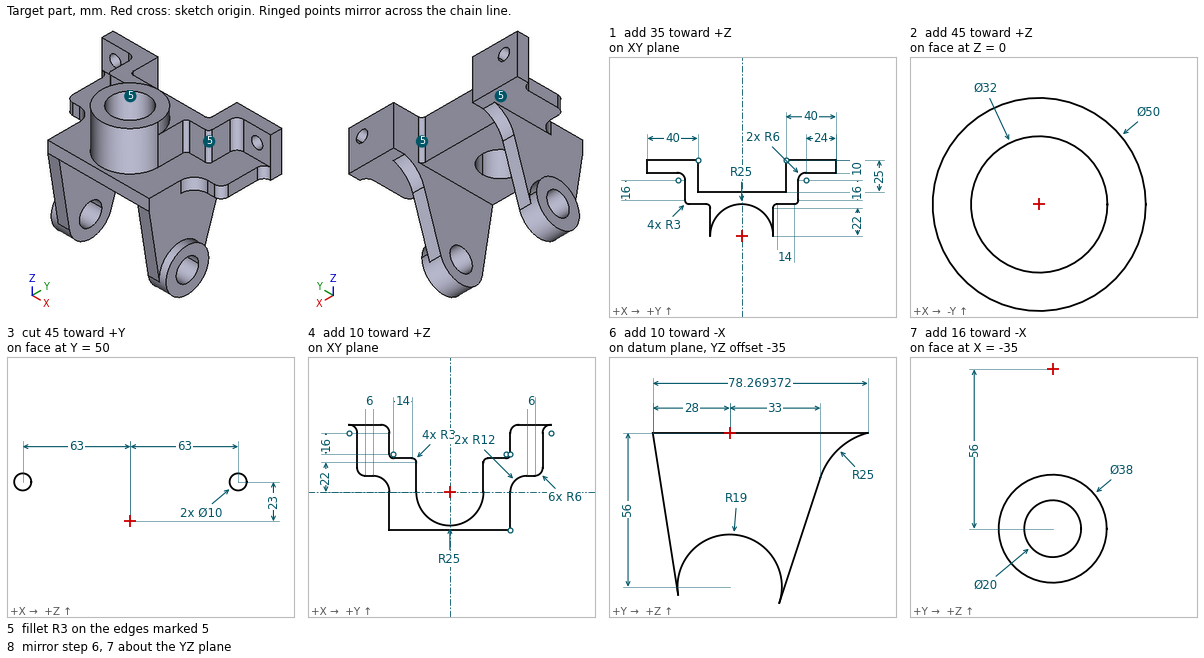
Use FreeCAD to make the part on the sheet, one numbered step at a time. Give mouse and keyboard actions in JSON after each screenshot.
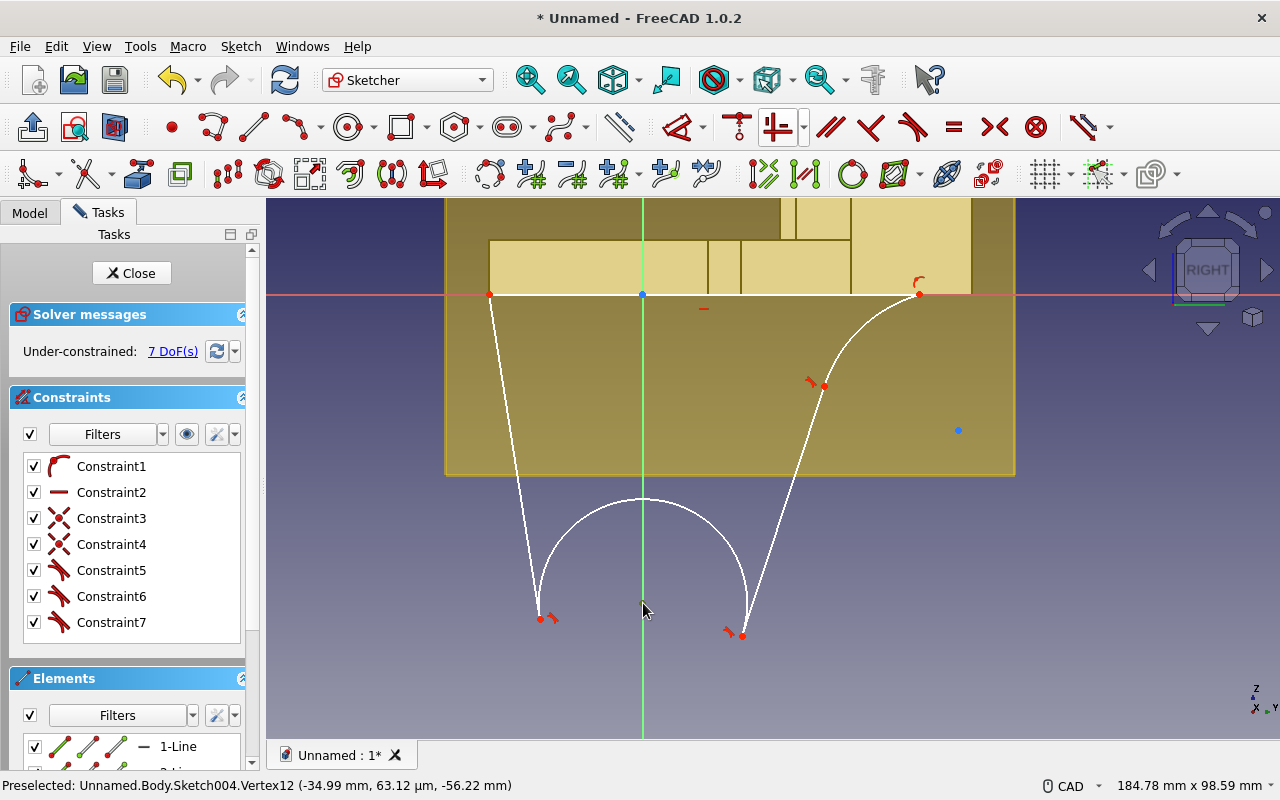
{"action": "left_click", "coordinate": [643, 676]}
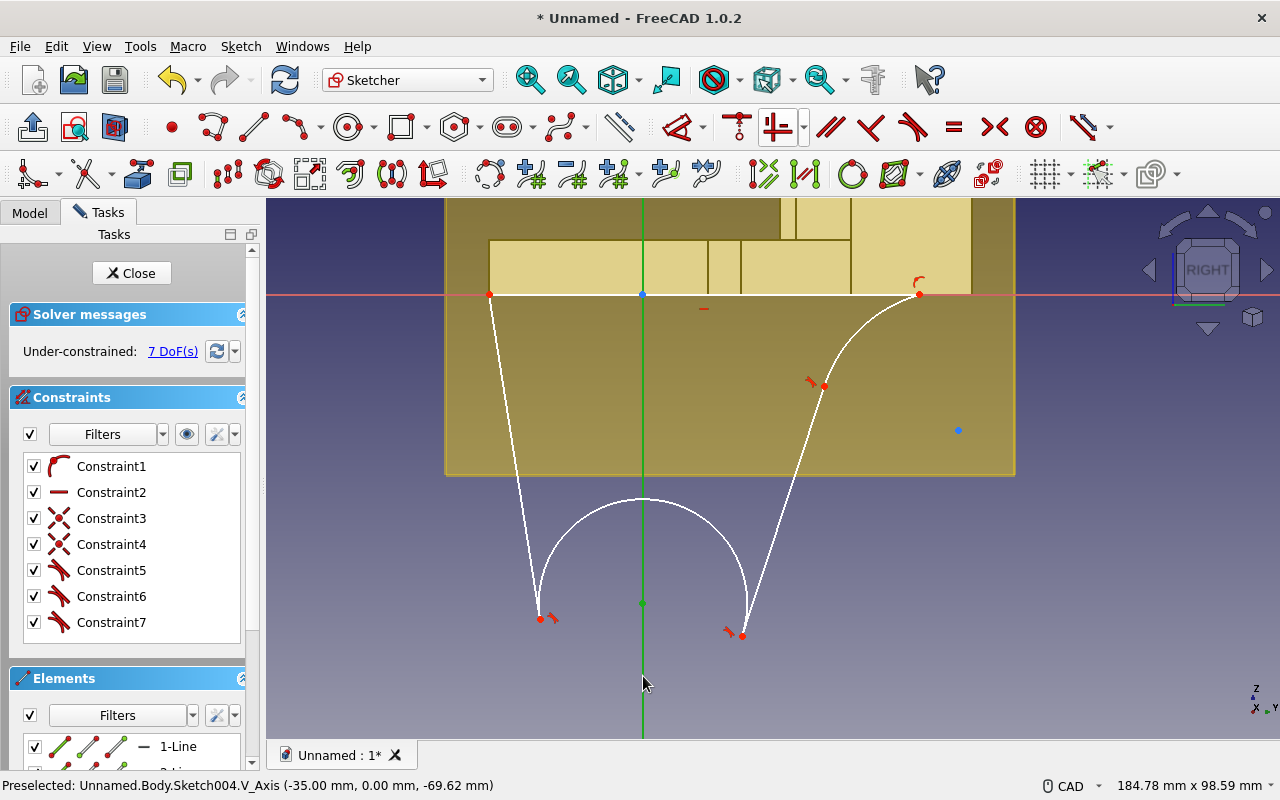
{"action": "left_click", "coordinate": [737, 128]}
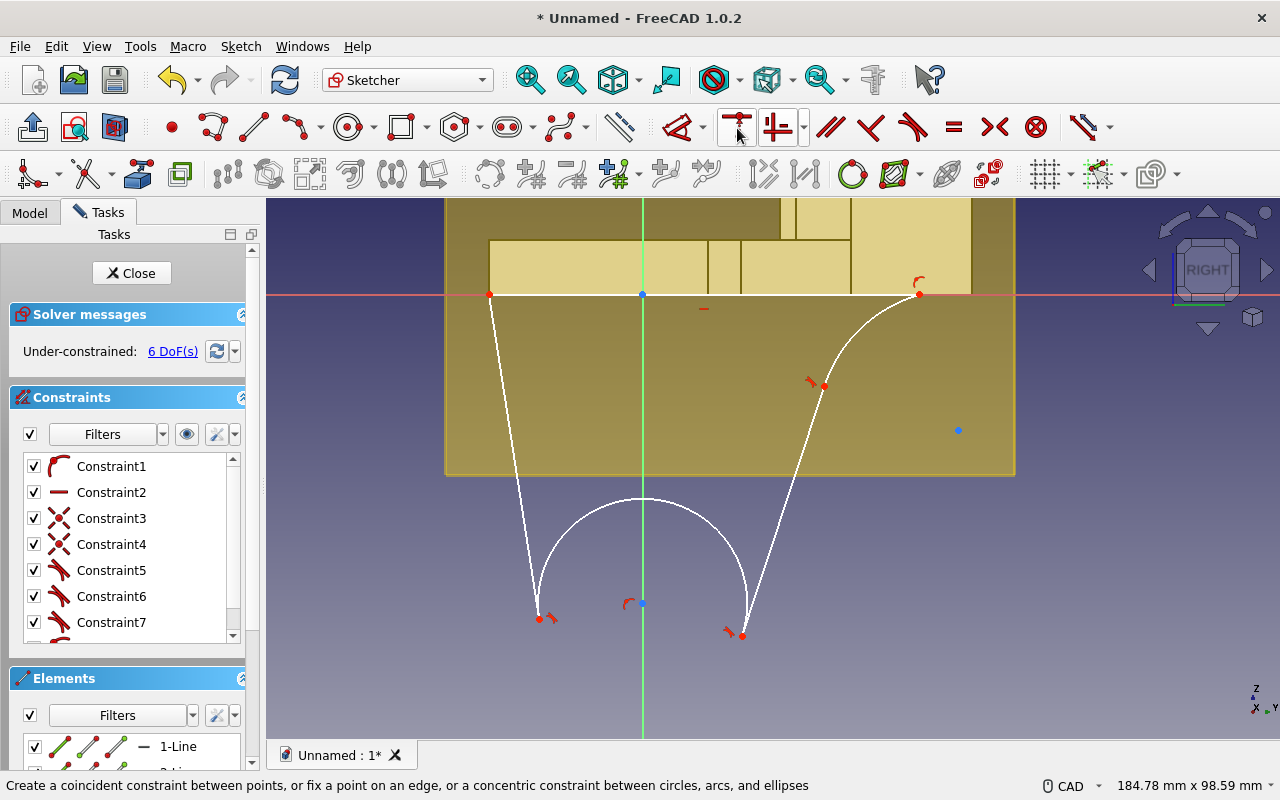
{"action": "left_click", "coordinate": [676, 128]}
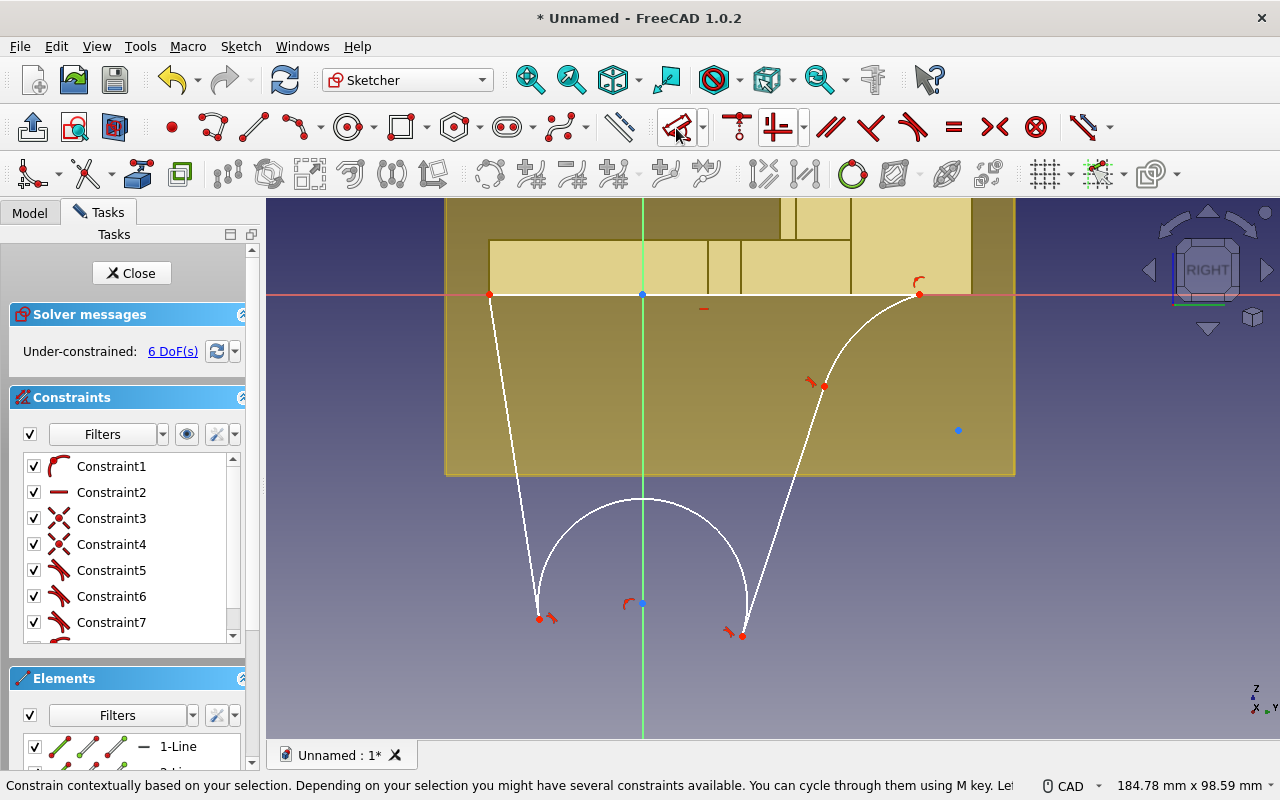
{"action": "left_click", "coordinate": [882, 312]}
{"action": "left_click", "coordinate": [946, 258]}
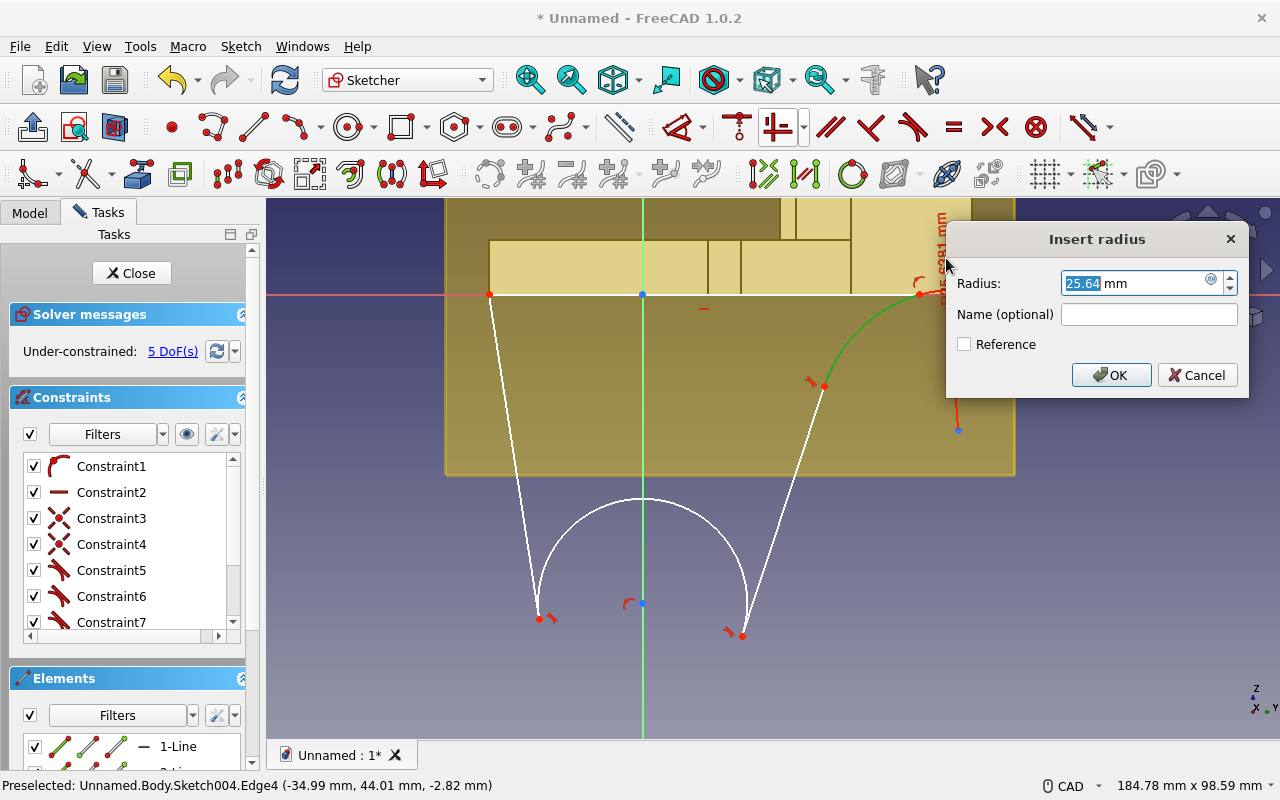
{"action": "type", "text": "25"}
{"action": "key", "text": "Return"}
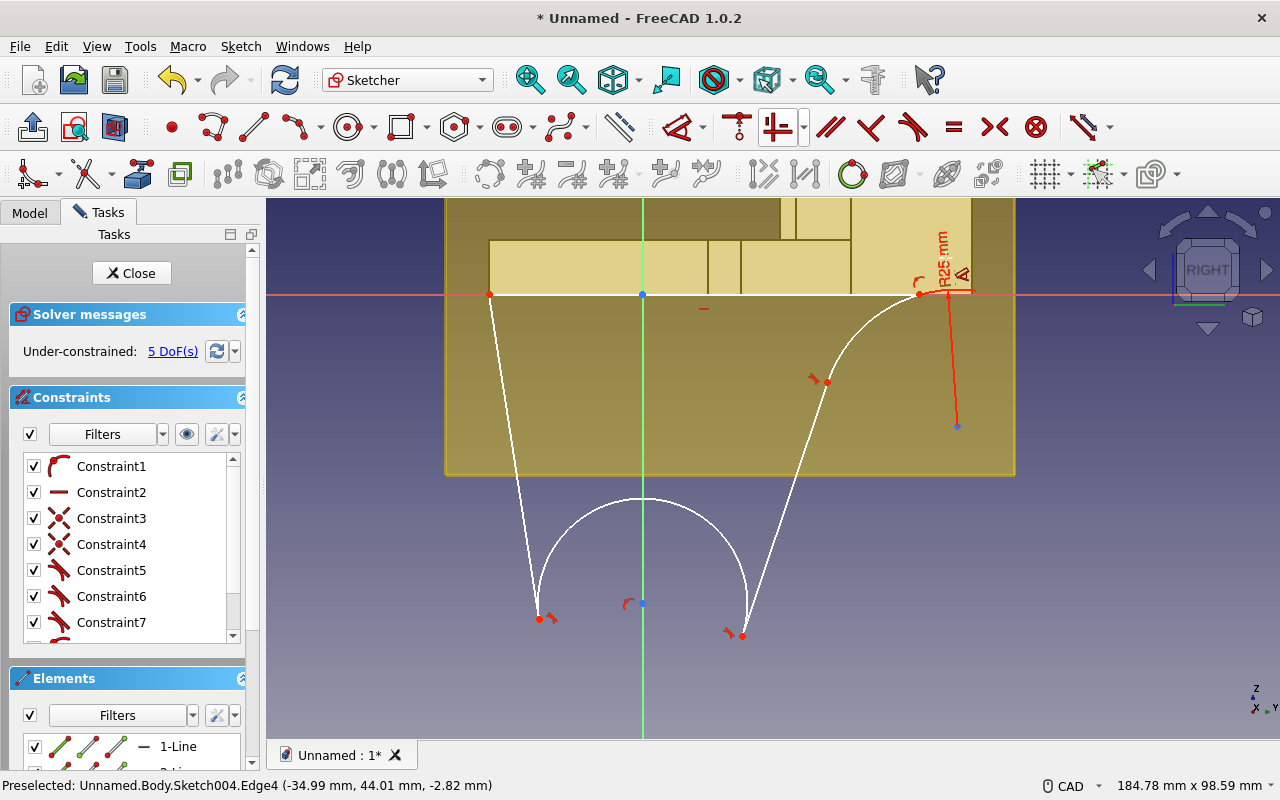
{"action": "left_click", "coordinate": [719, 531]}
{"action": "left_click", "coordinate": [742, 509]}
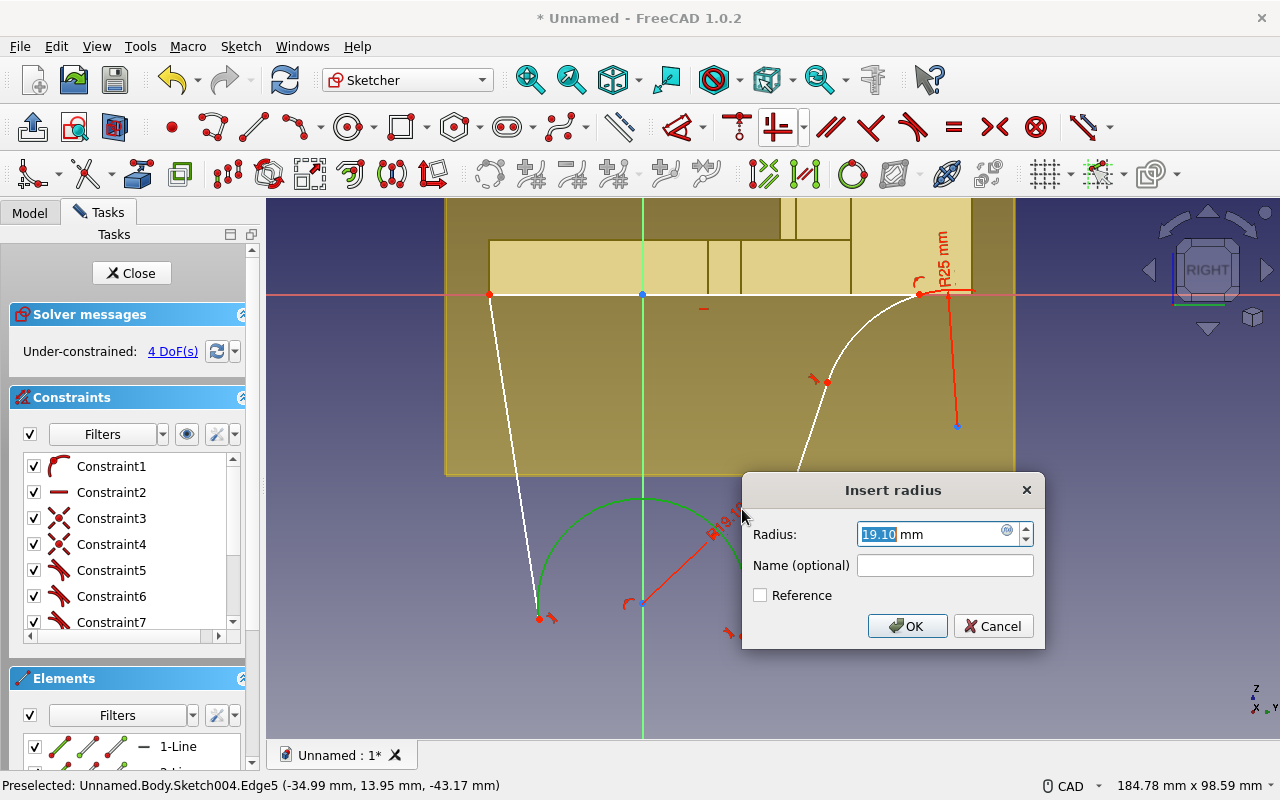
{"action": "type", "text": "19"}
{"action": "key", "text": "Return"}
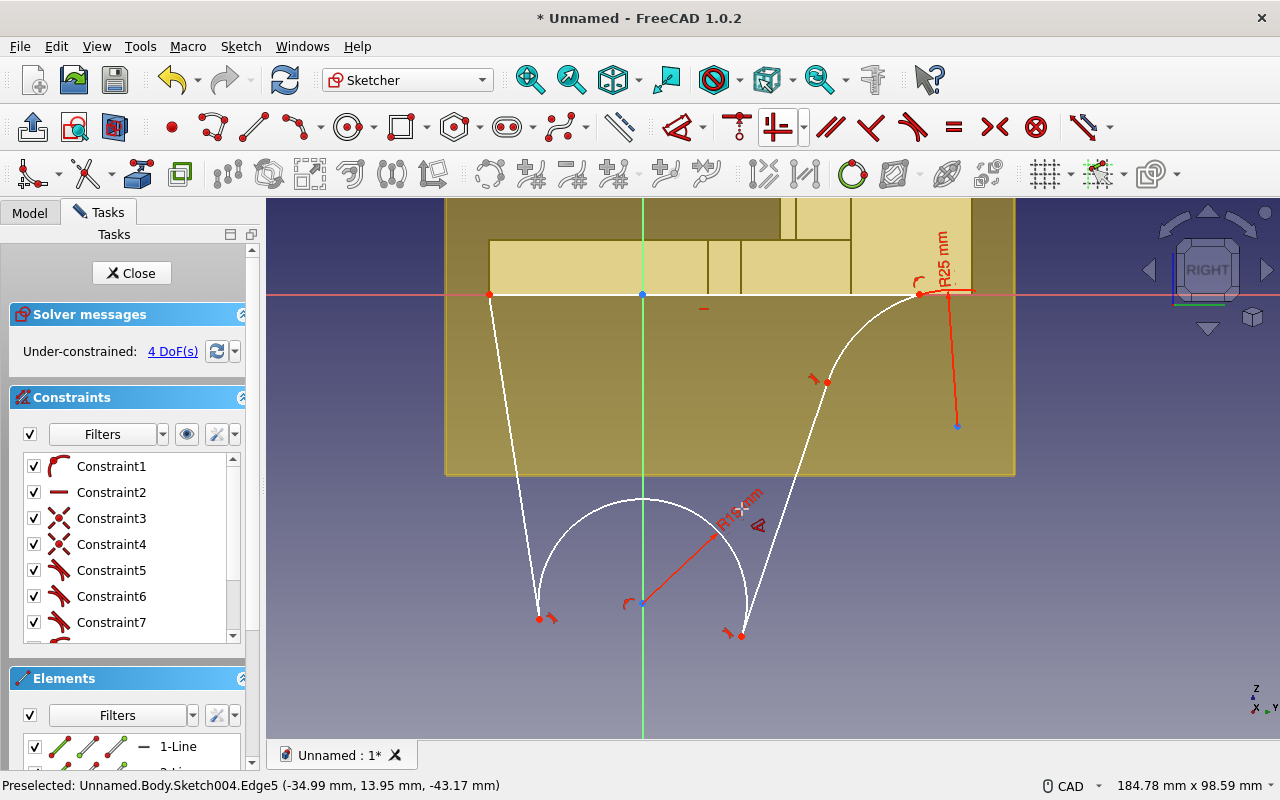
{"action": "left_click", "coordinate": [828, 383]}
{"action": "left_click", "coordinate": [735, 261]}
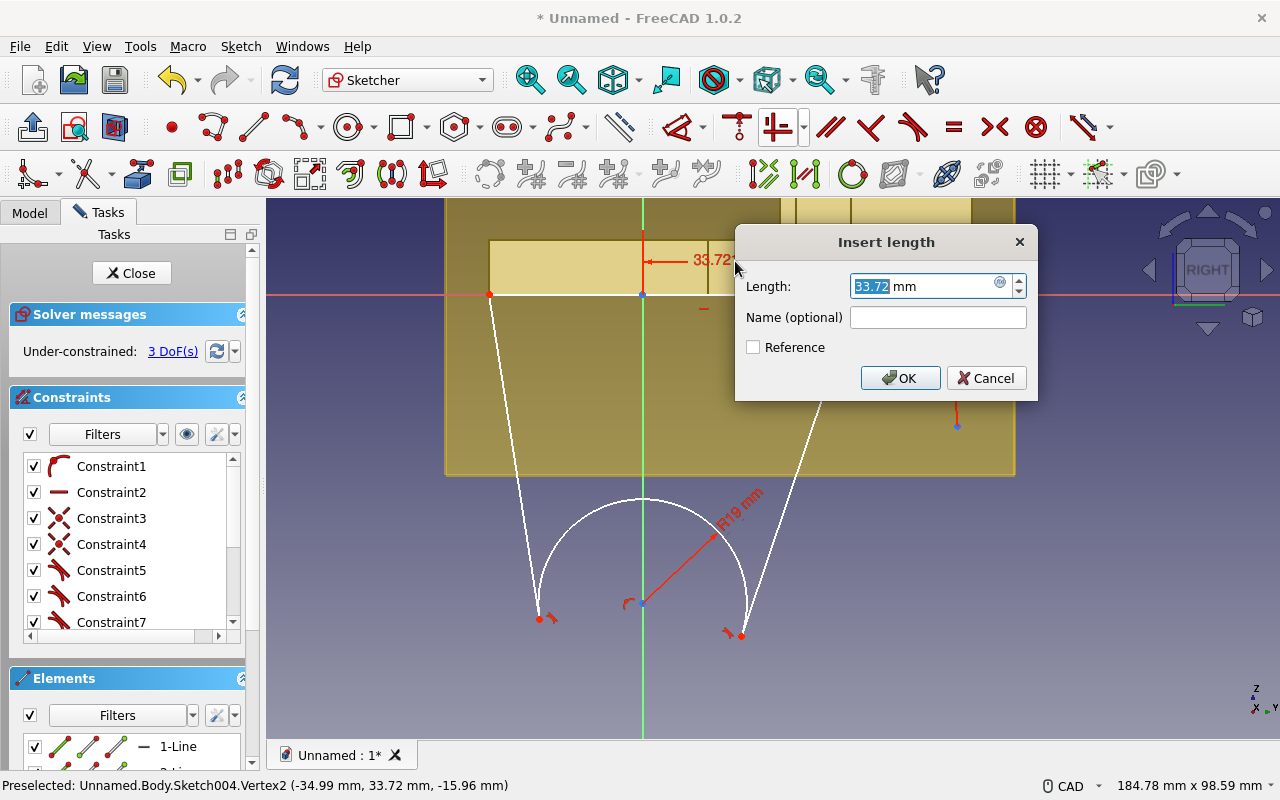
{"action": "type", "text": "33"}
{"action": "key", "text": "Return"}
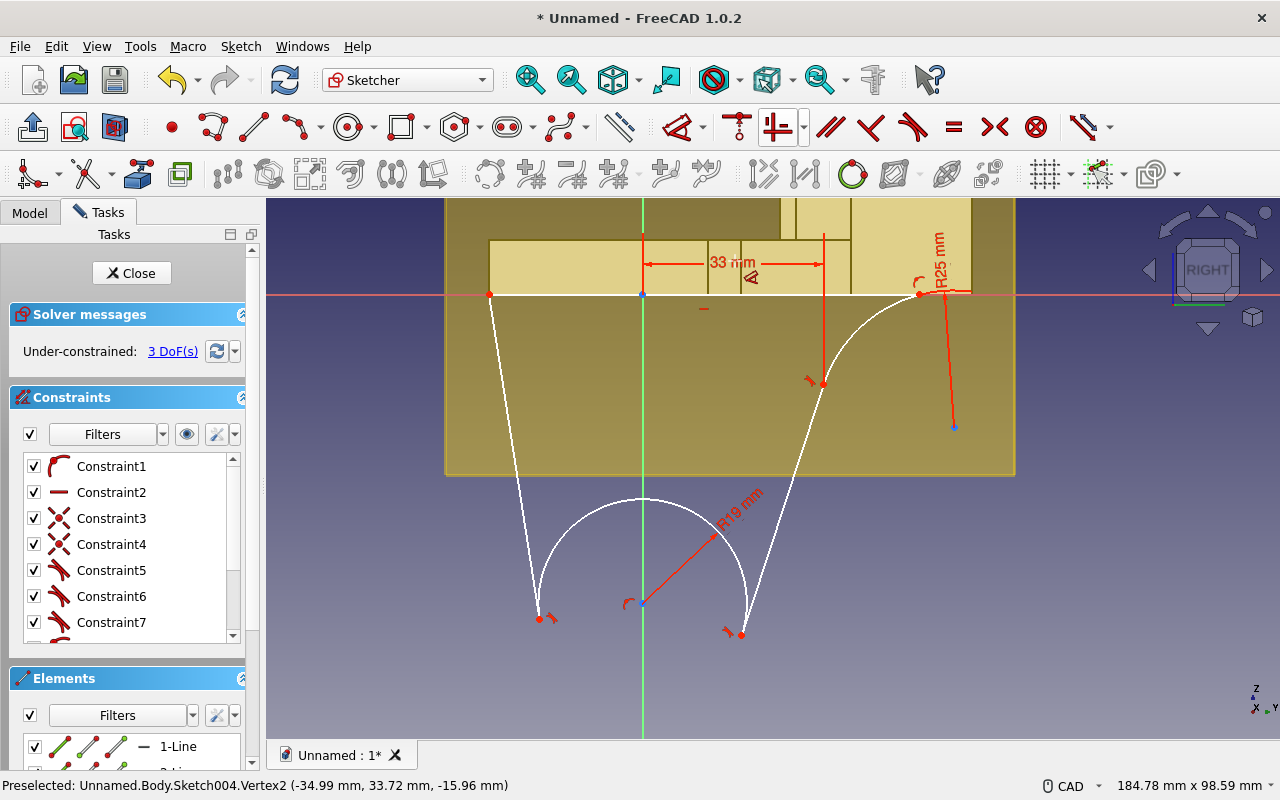
{"action": "left_click", "coordinate": [489, 295]}
{"action": "left_click", "coordinate": [566, 261]}